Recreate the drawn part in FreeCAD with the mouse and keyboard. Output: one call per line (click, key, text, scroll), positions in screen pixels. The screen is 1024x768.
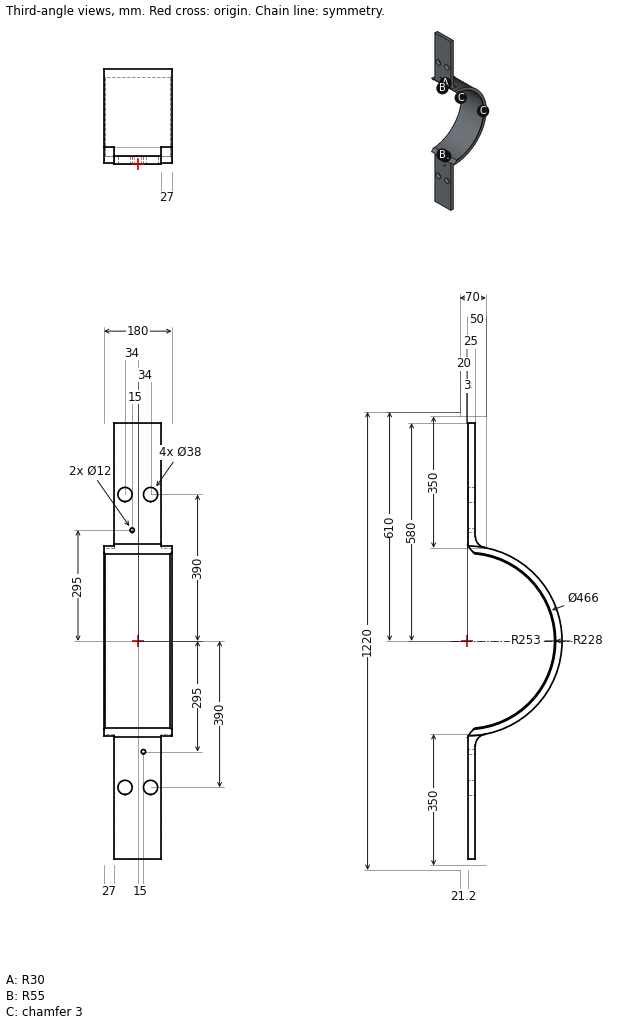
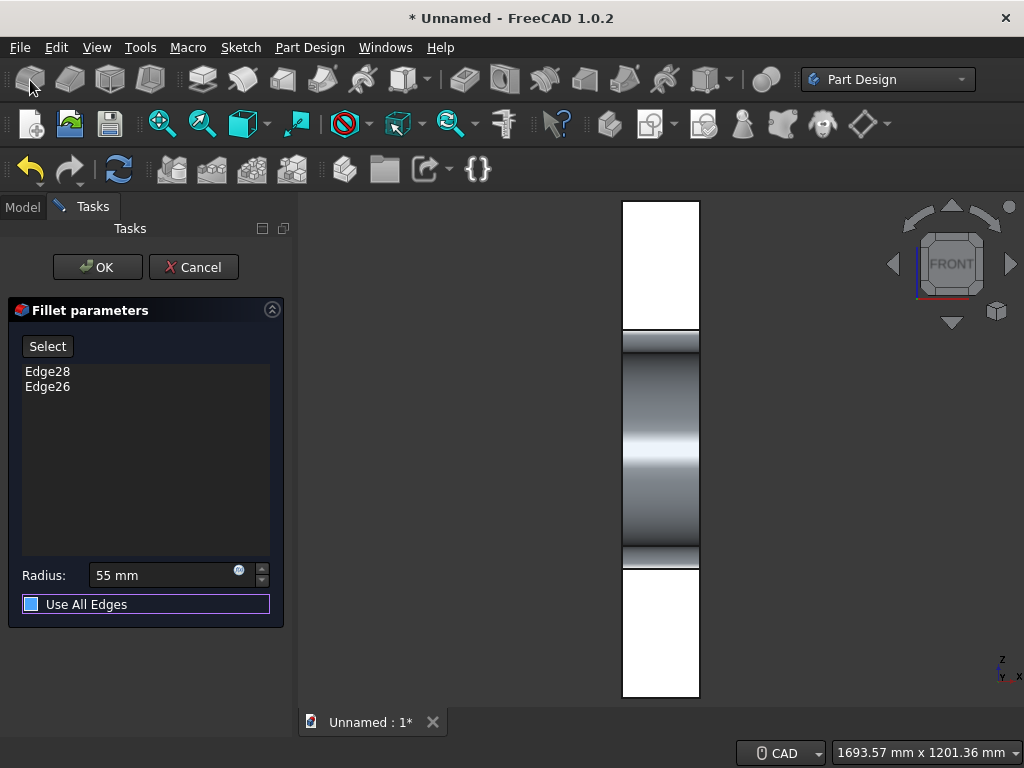
click(98, 267)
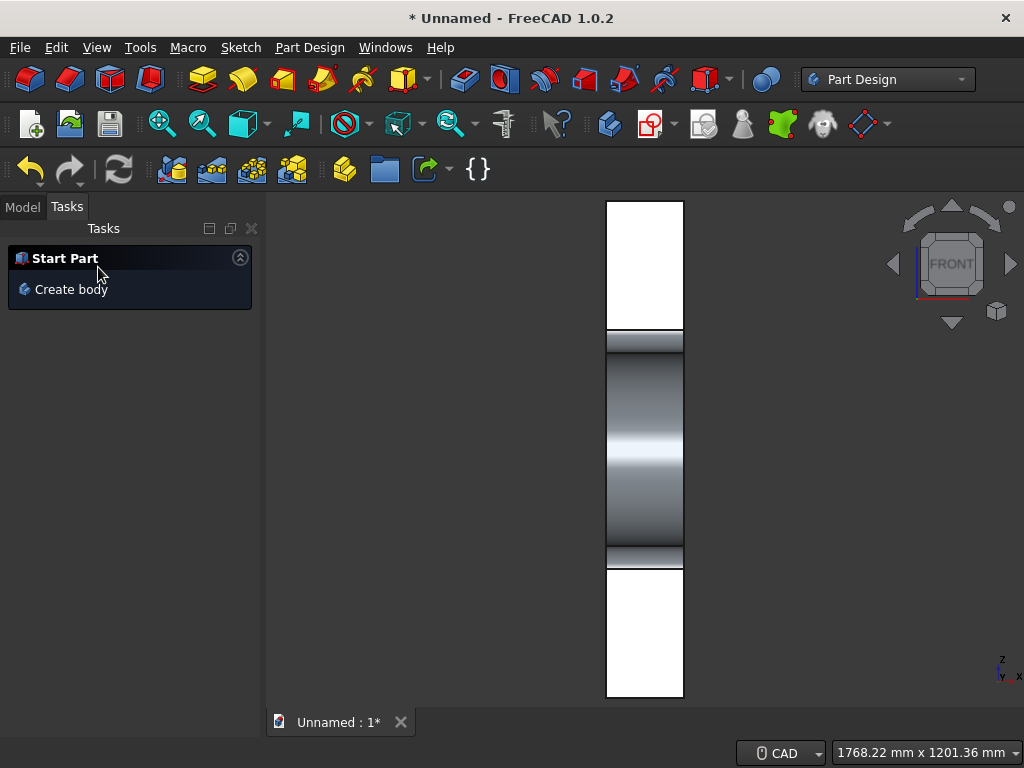
click(650, 124)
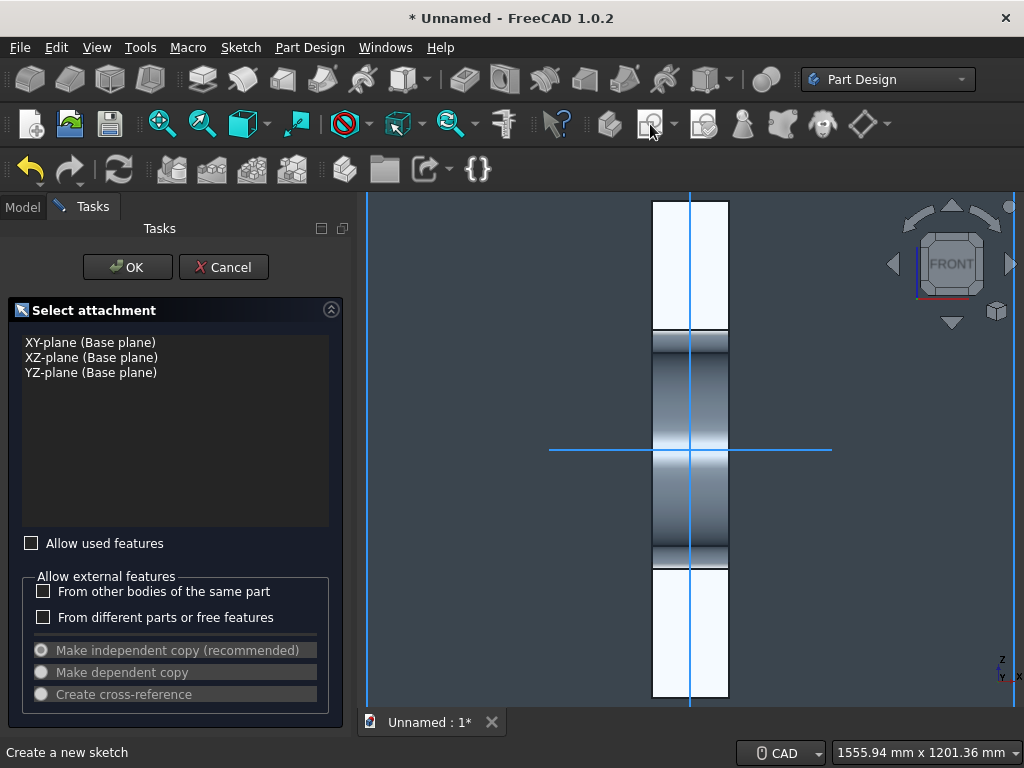
click(82, 372)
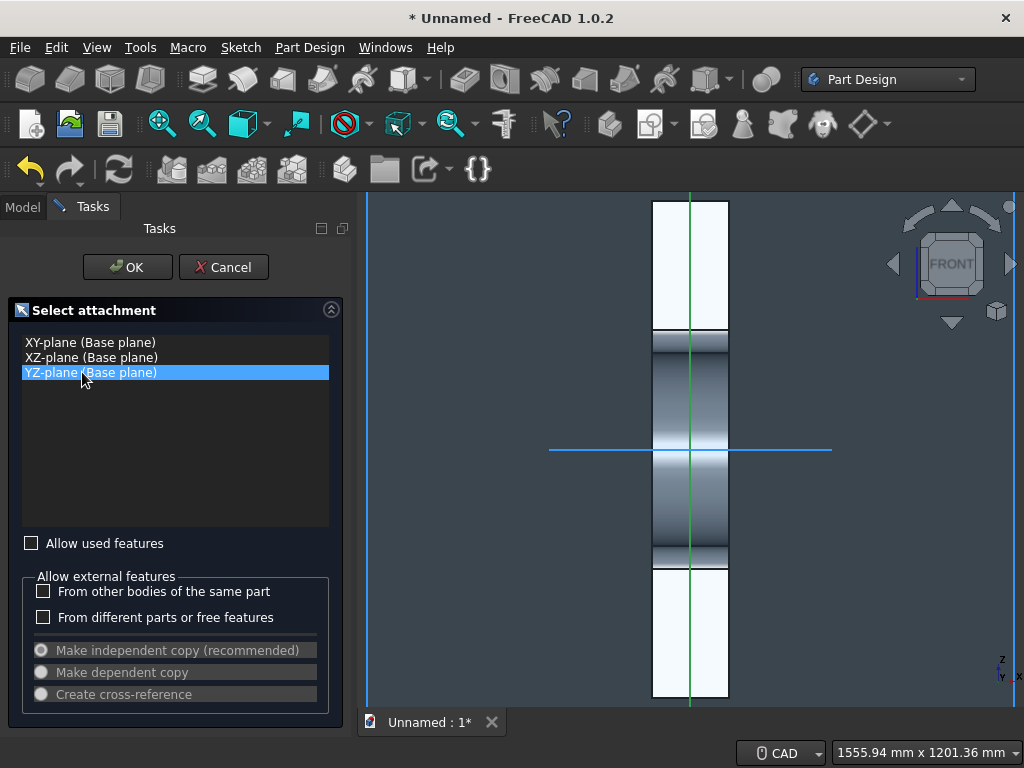
click(128, 267)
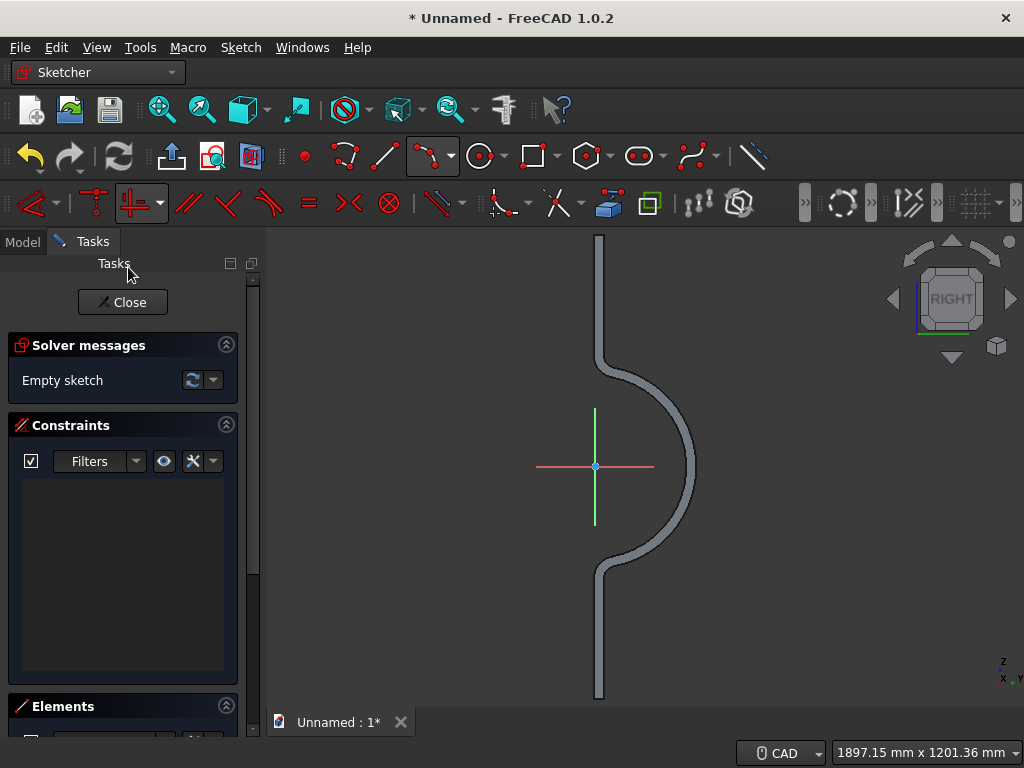
click(252, 156)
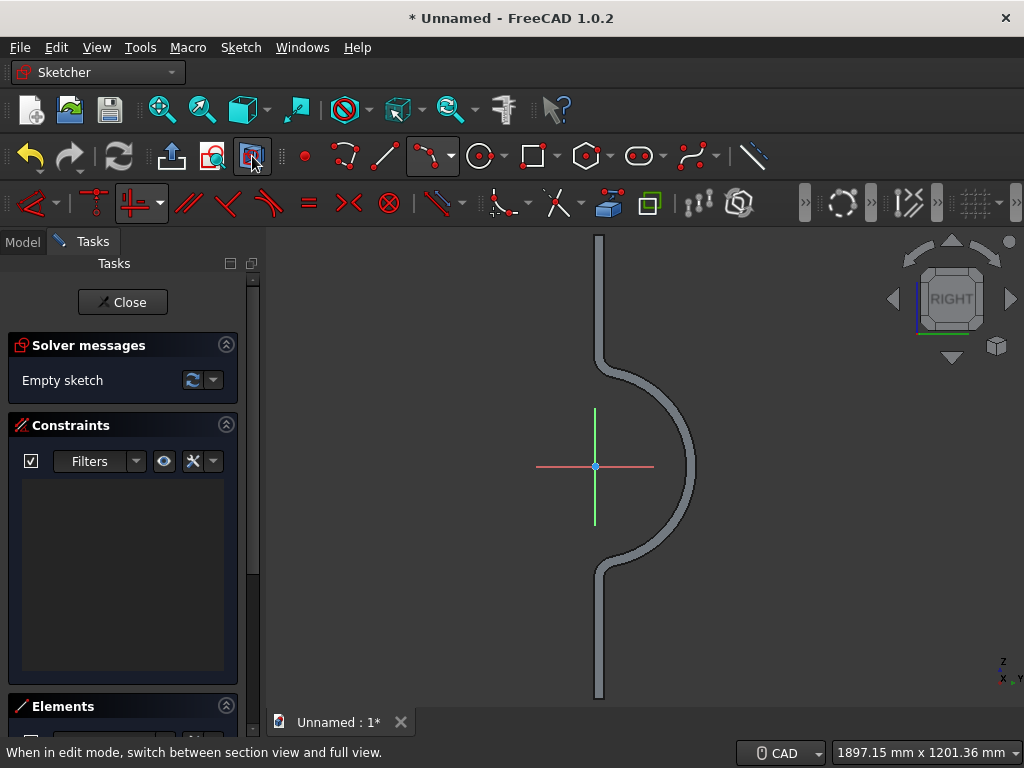
scroll(633, 467, up, 2)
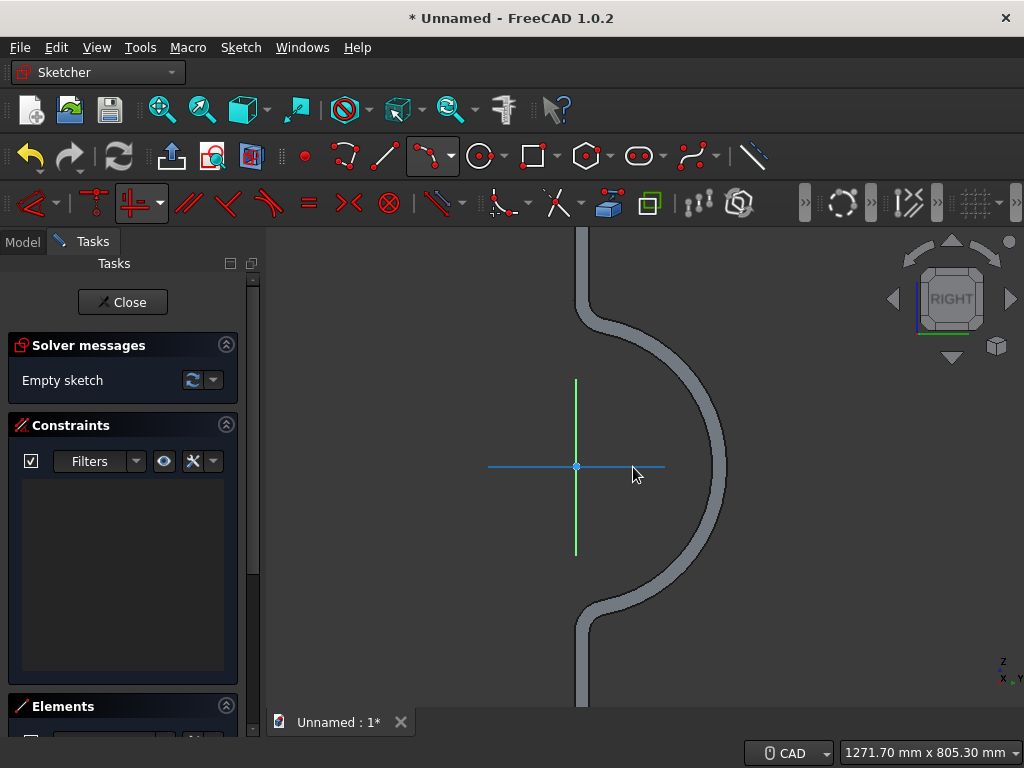
click(480, 156)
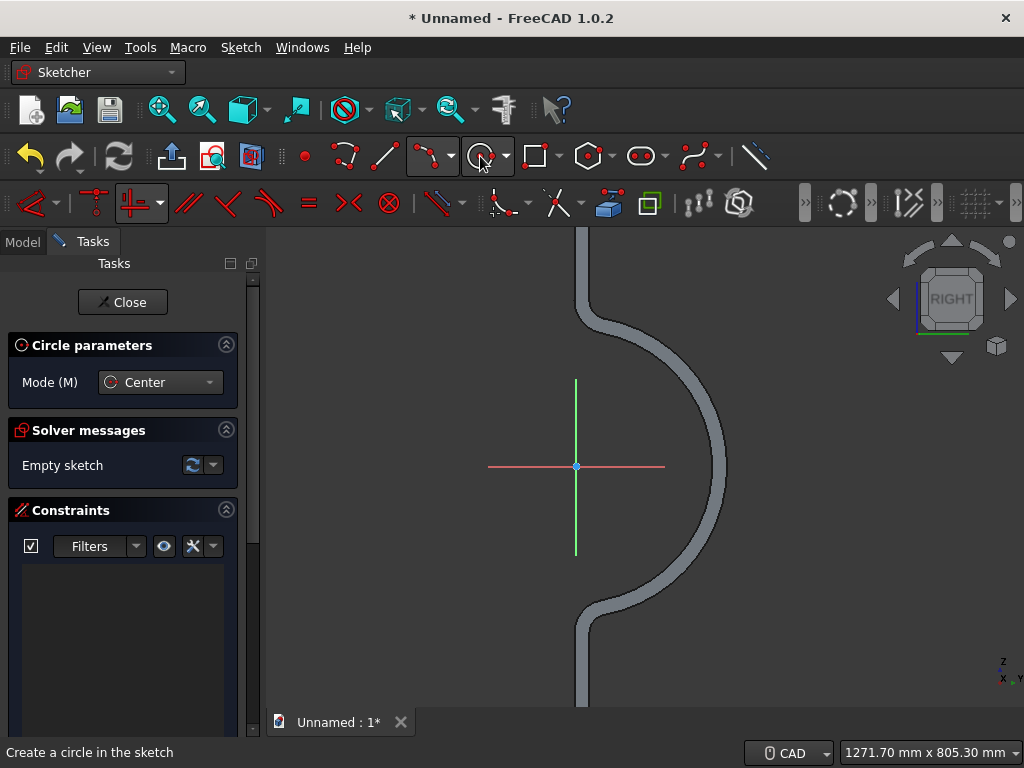
click(576, 467)
click(675, 369)
key(Escape)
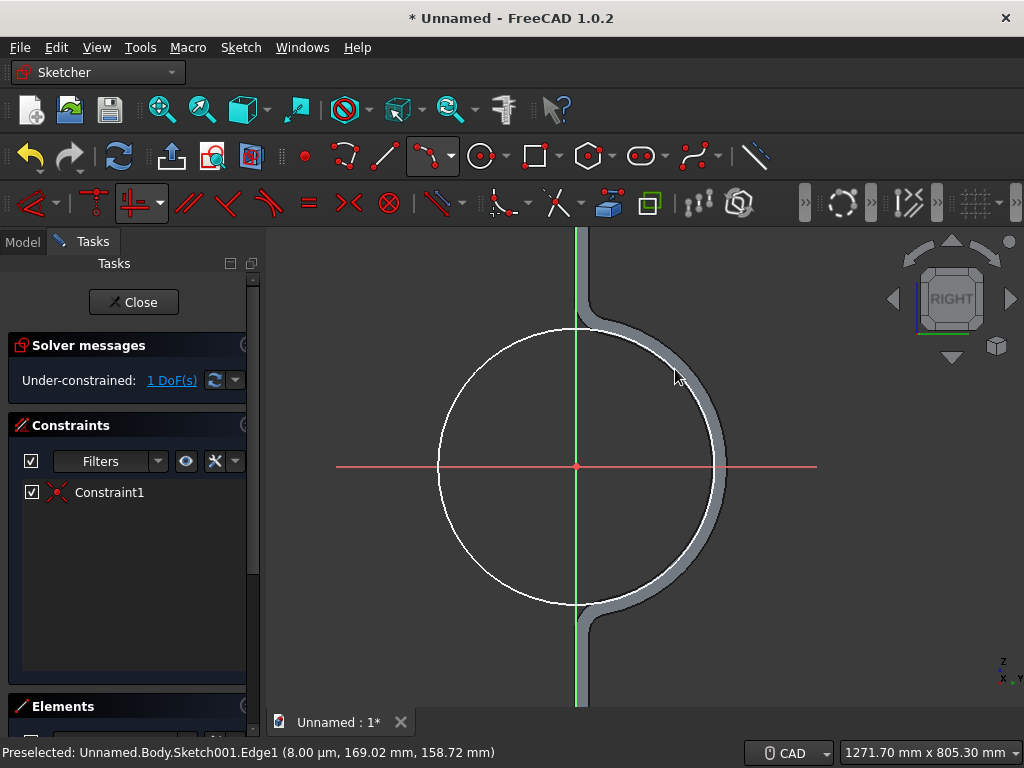
click(32, 204)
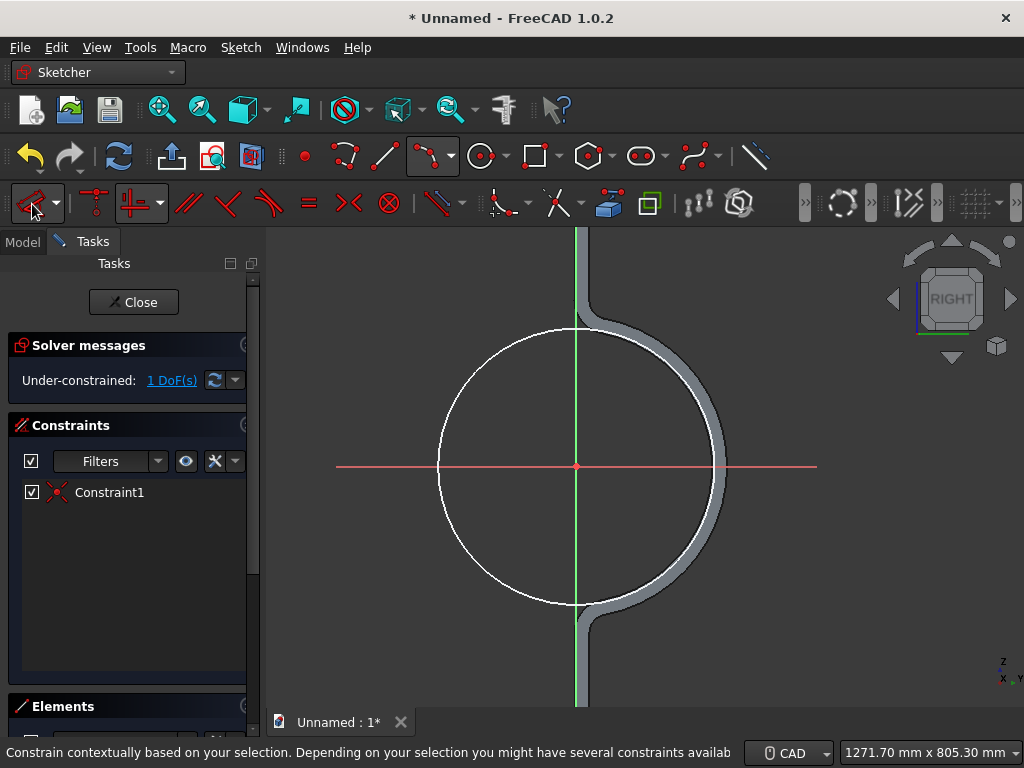
click(674, 369)
click(697, 346)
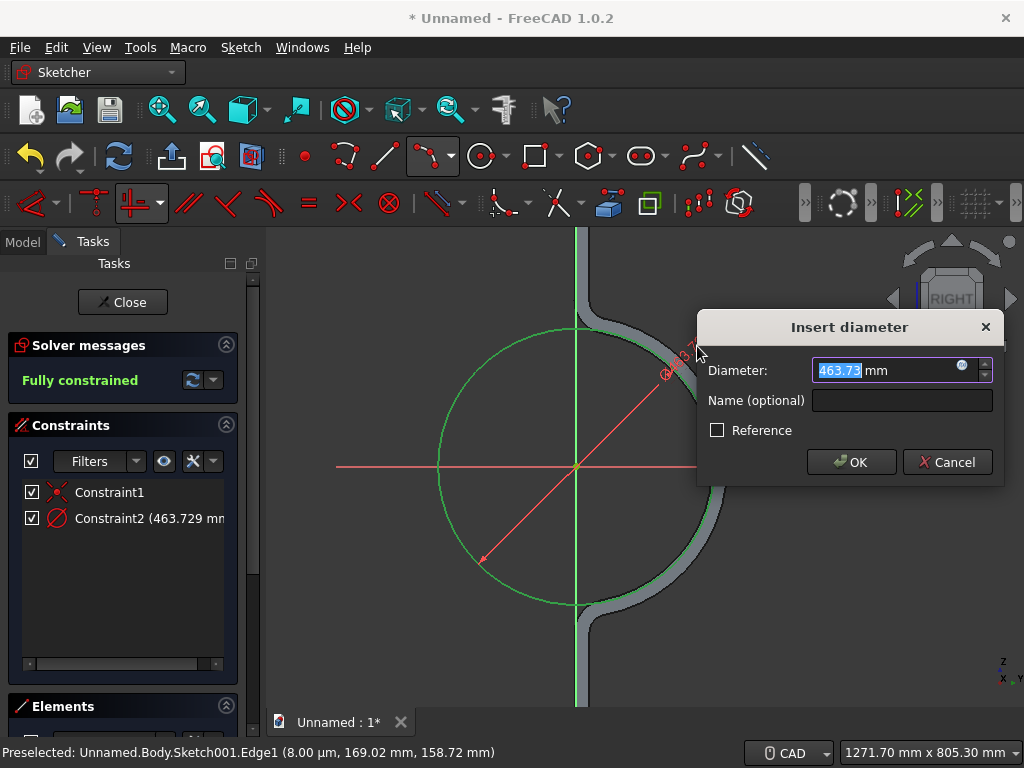
text(466)
key(Return)
key(Escape)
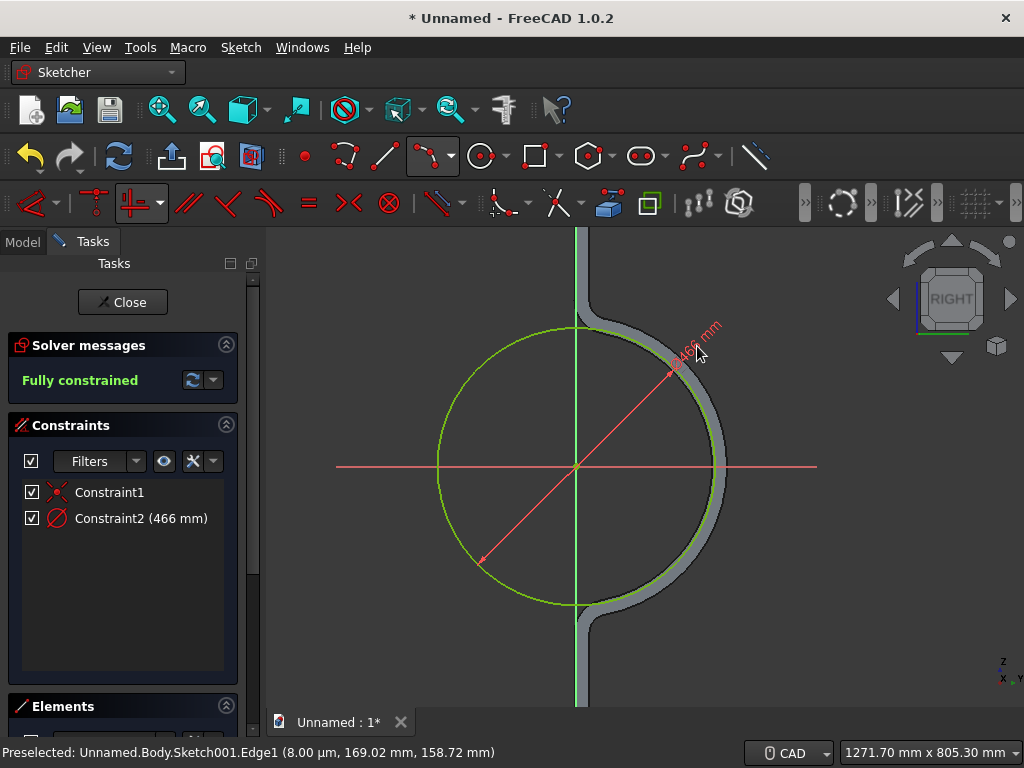
click(123, 302)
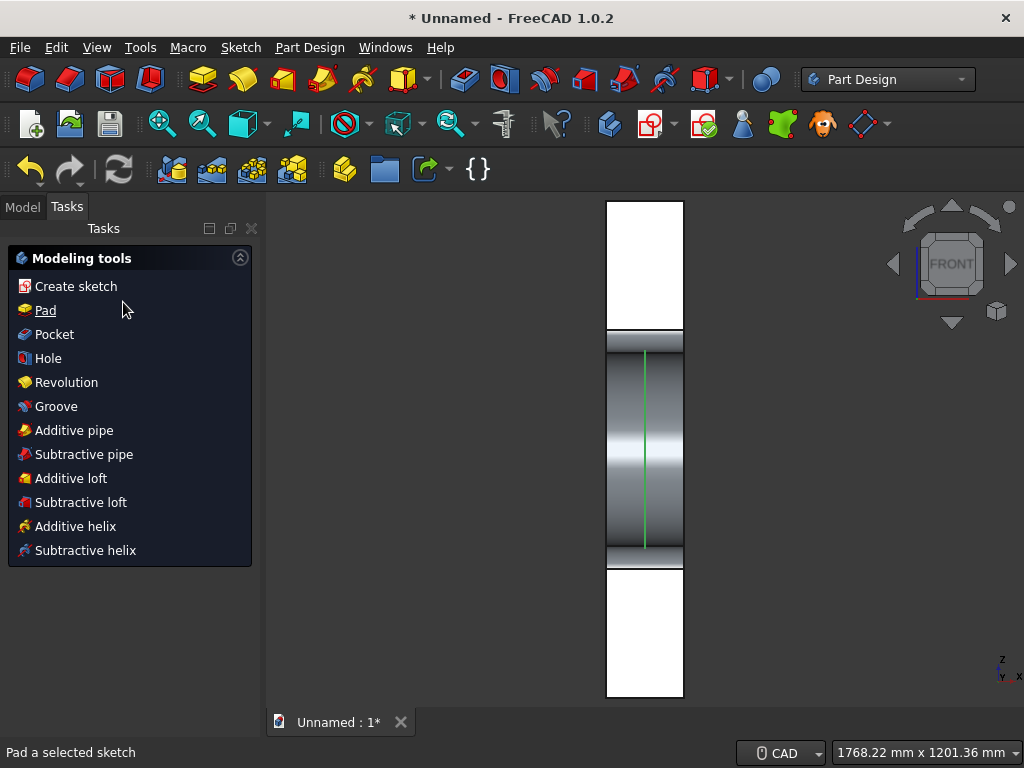
click(466, 80)